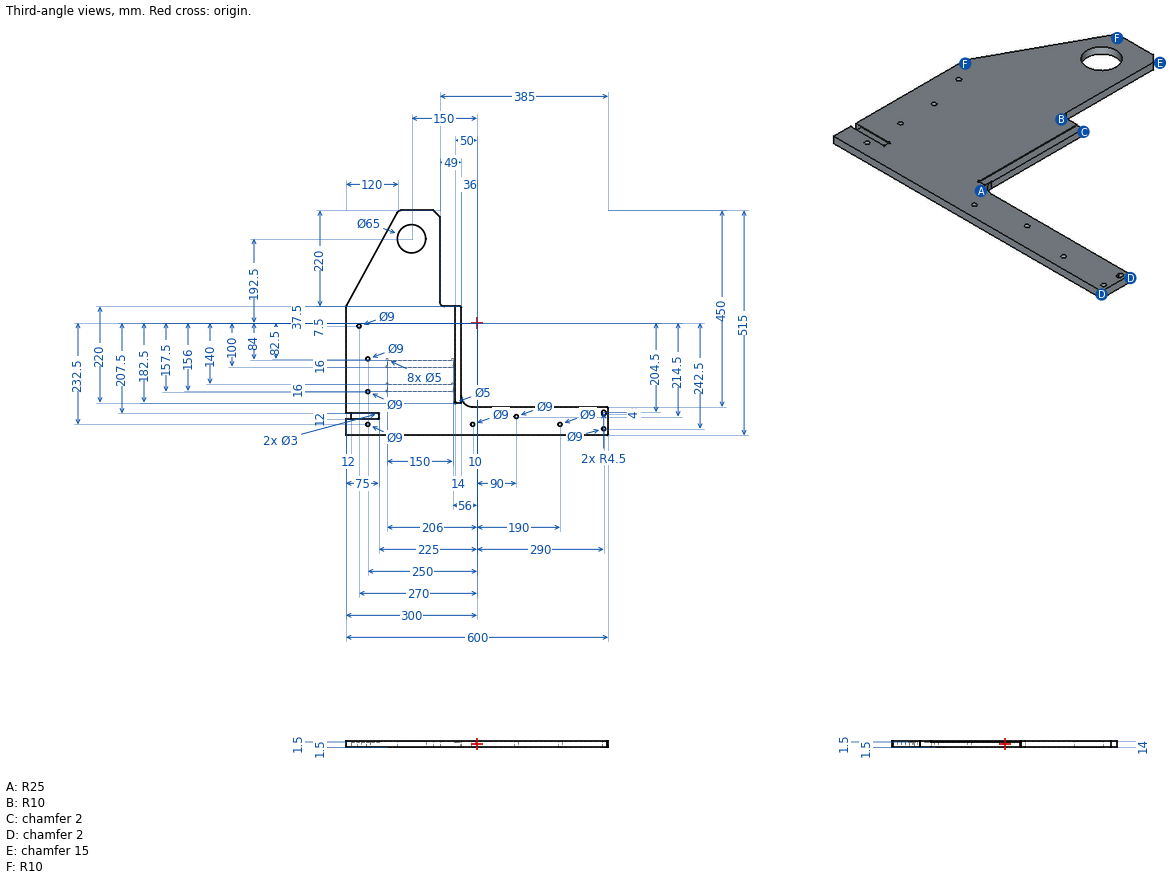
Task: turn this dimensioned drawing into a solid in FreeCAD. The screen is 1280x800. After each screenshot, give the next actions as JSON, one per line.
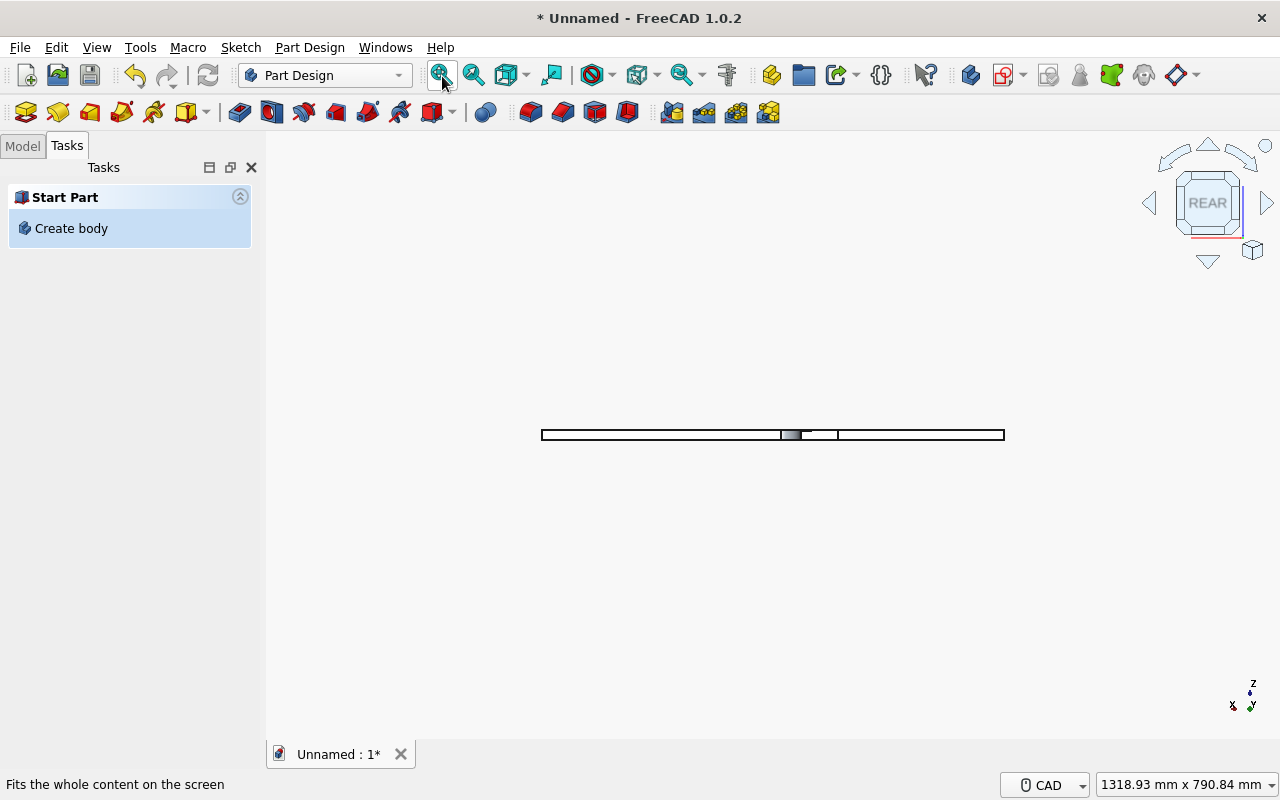
{"action": "scroll", "coordinate": [838, 434], "scroll_direction": "up", "scroll_amount": 7}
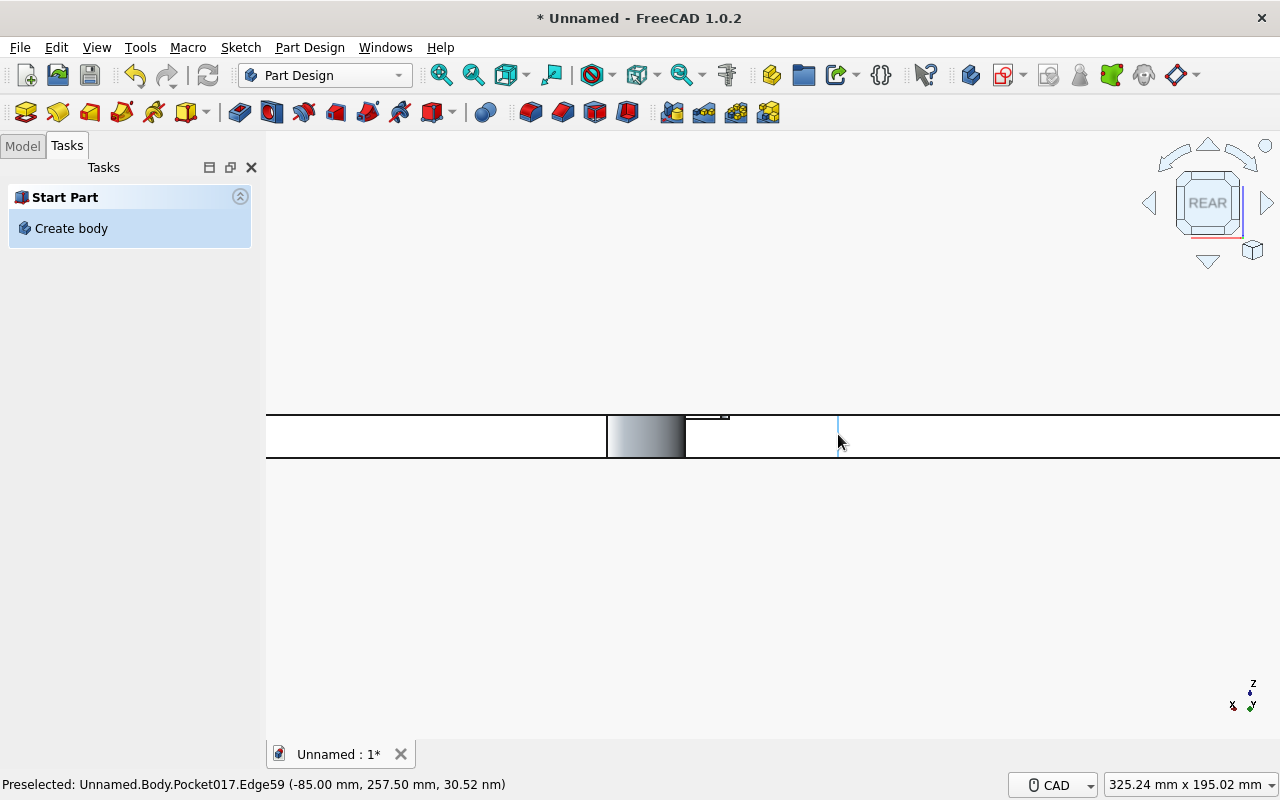
{"action": "left_click", "coordinate": [442, 76]}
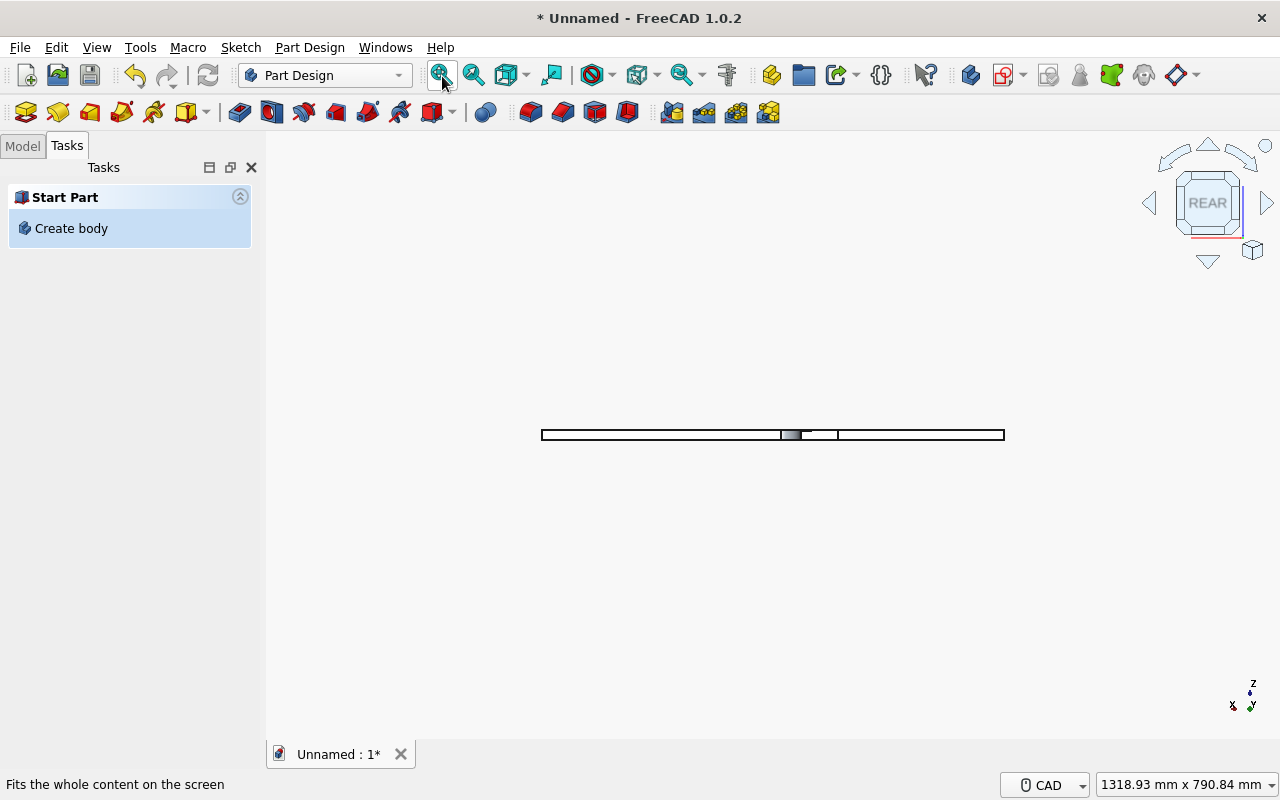
{"action": "key", "text": "6"}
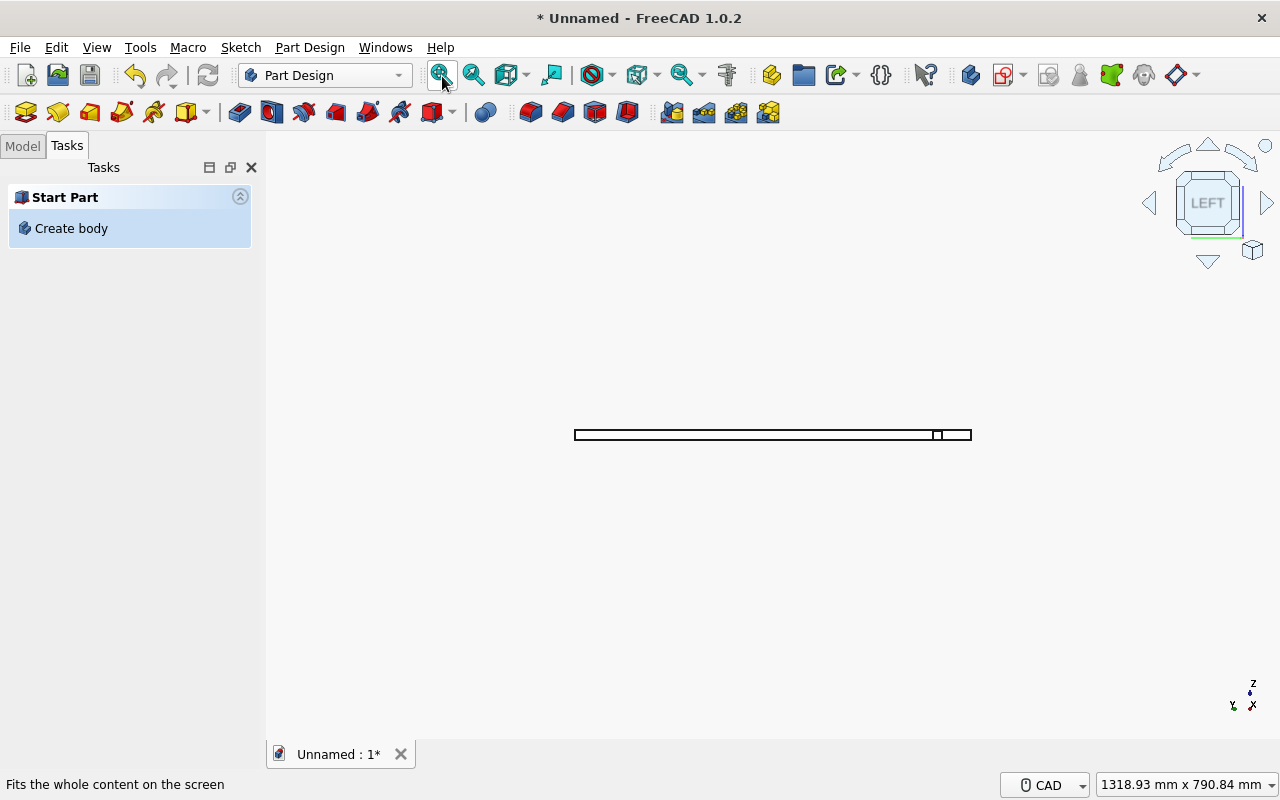
{"action": "left_click", "coordinate": [442, 76]}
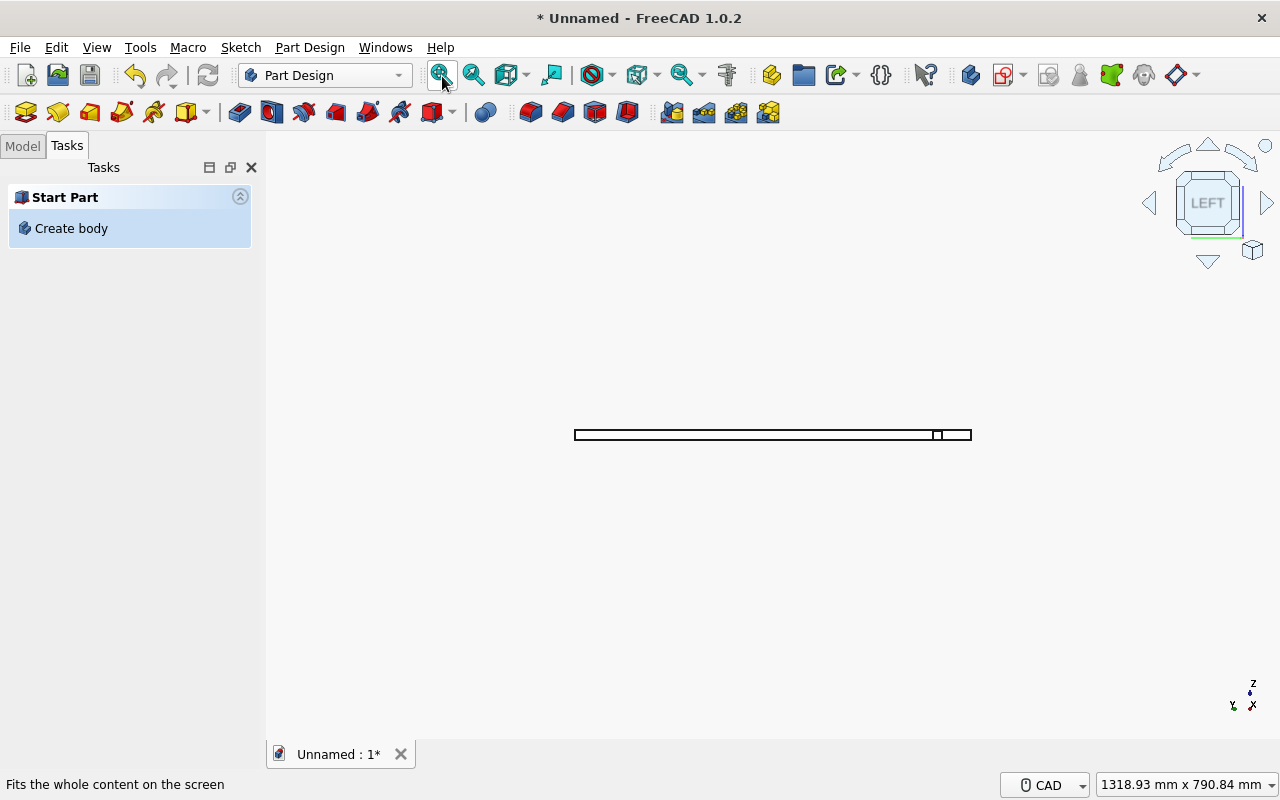
{"action": "scroll", "coordinate": [744, 434], "scroll_direction": "up", "scroll_amount": 7}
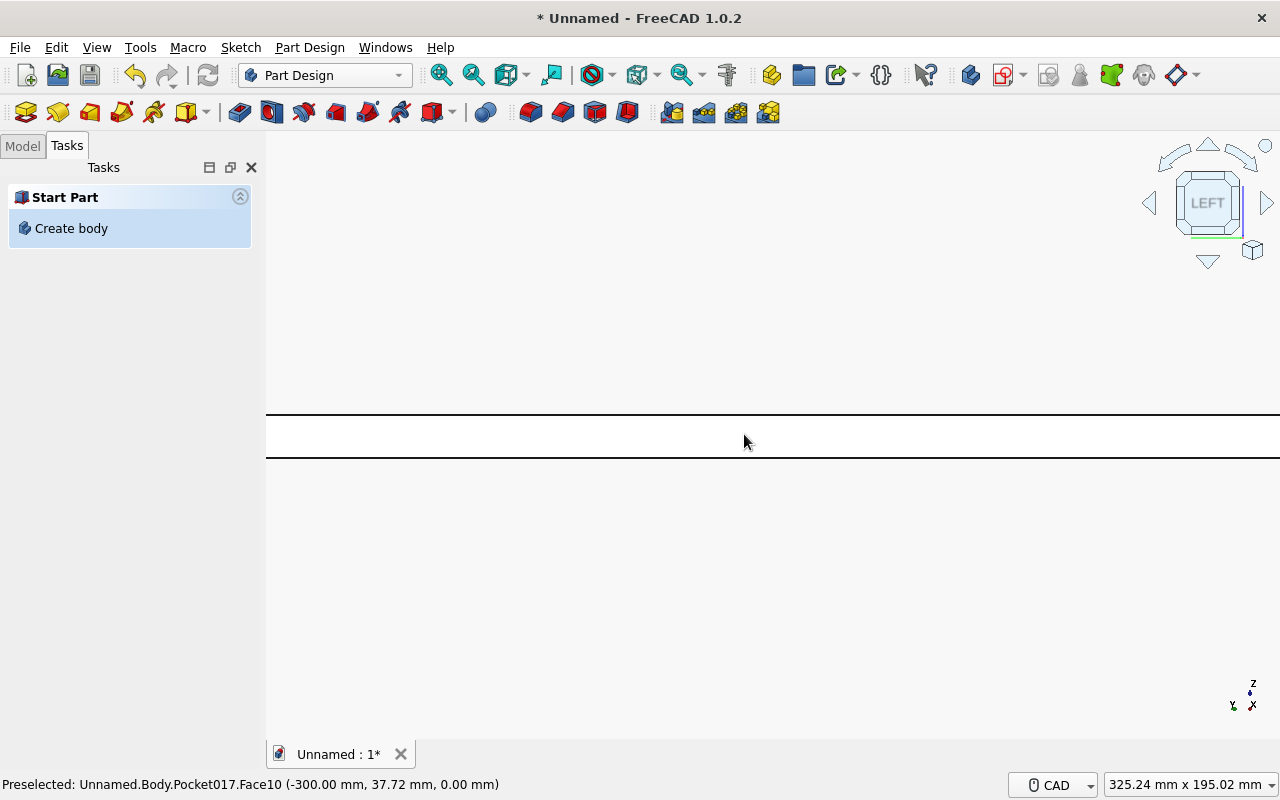
{"action": "left_click", "coordinate": [442, 76]}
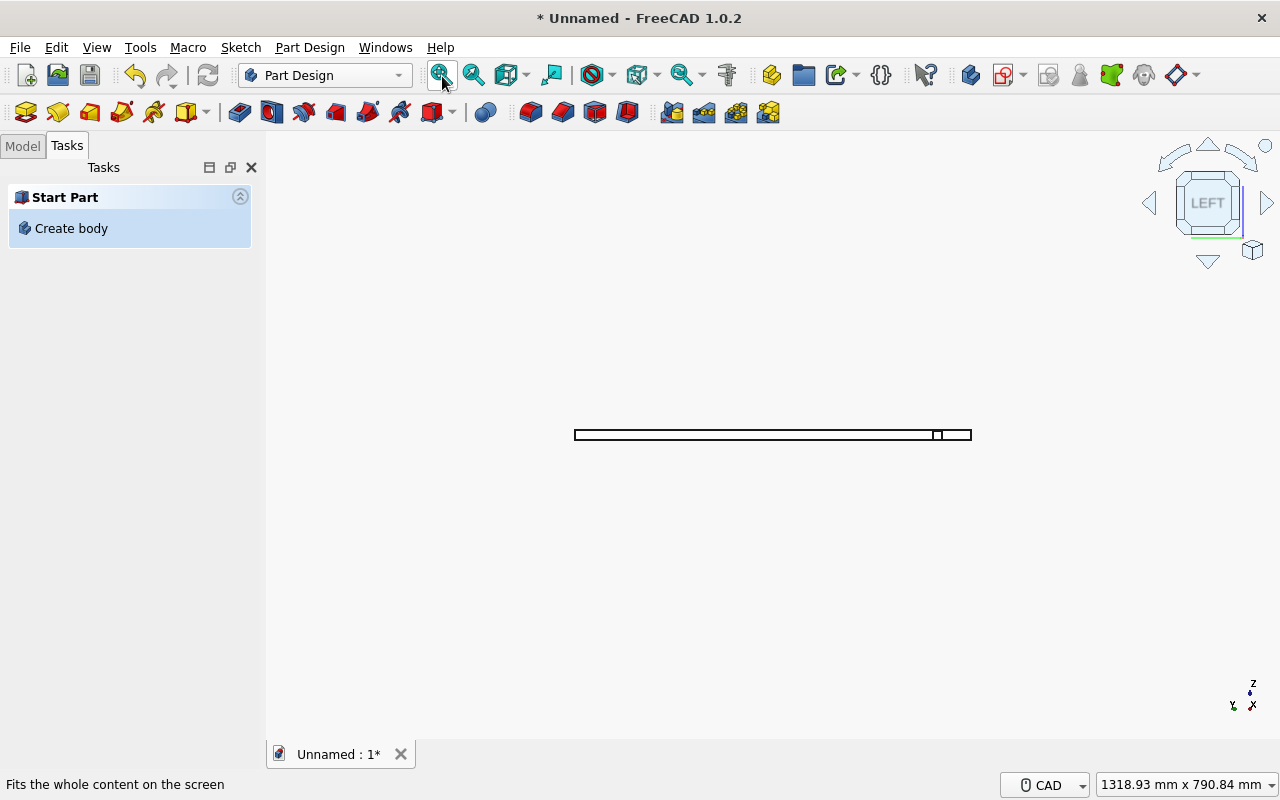
{"action": "key", "text": "v 3"}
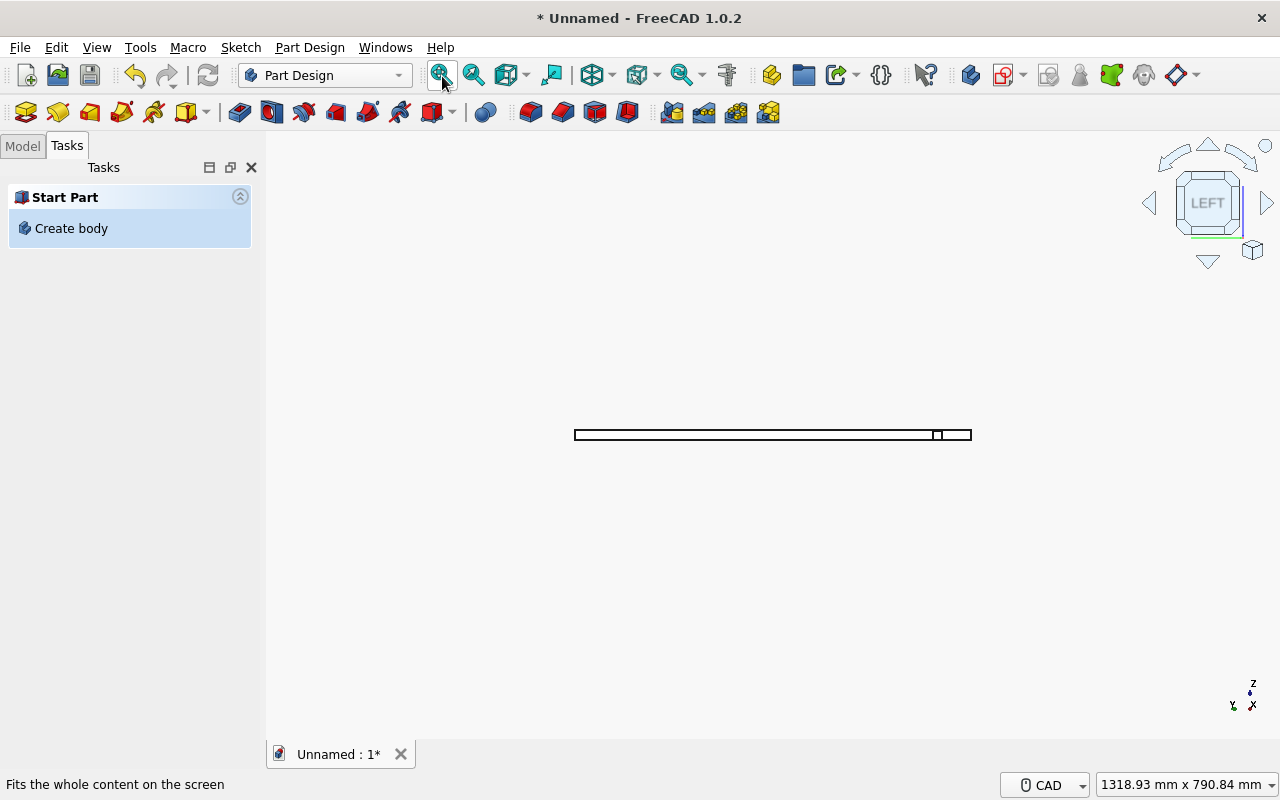
{"action": "key", "text": "0"}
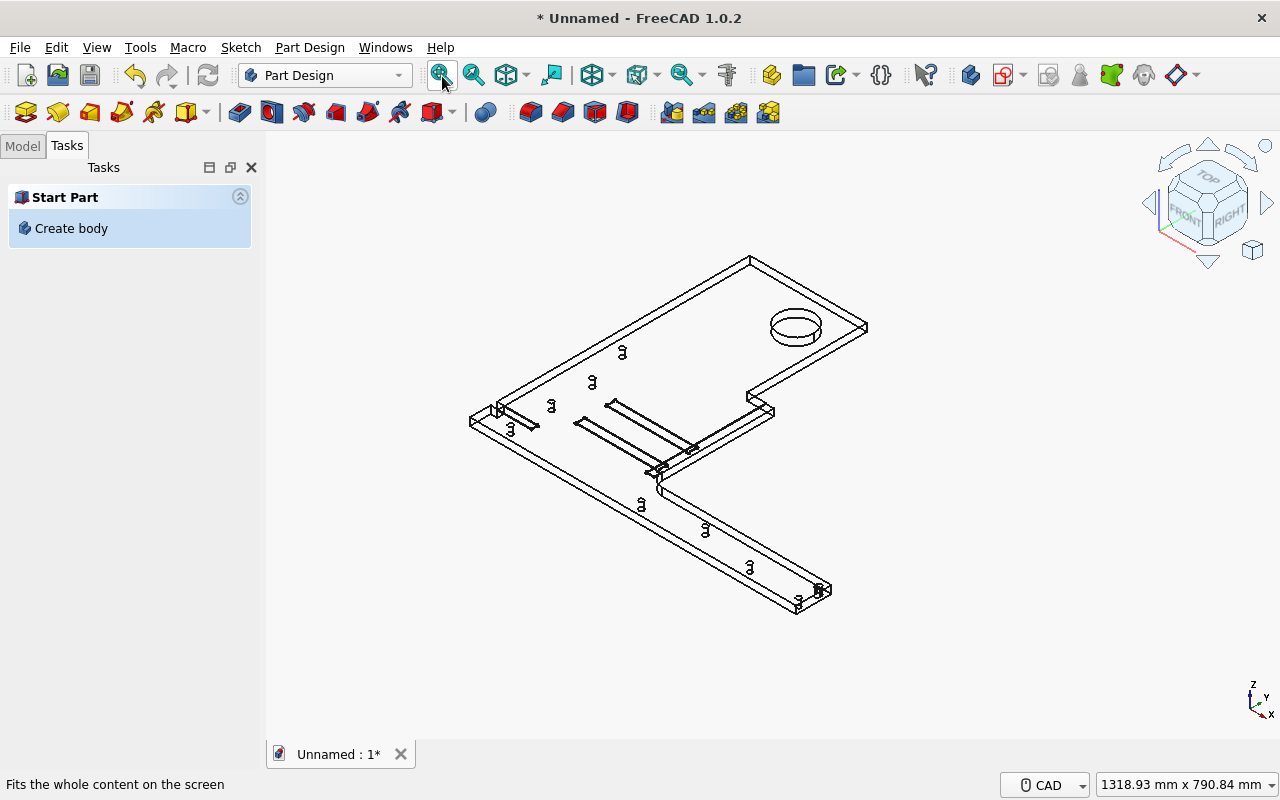
{"action": "scroll", "coordinate": [747, 396], "scroll_direction": "up", "scroll_amount": 7}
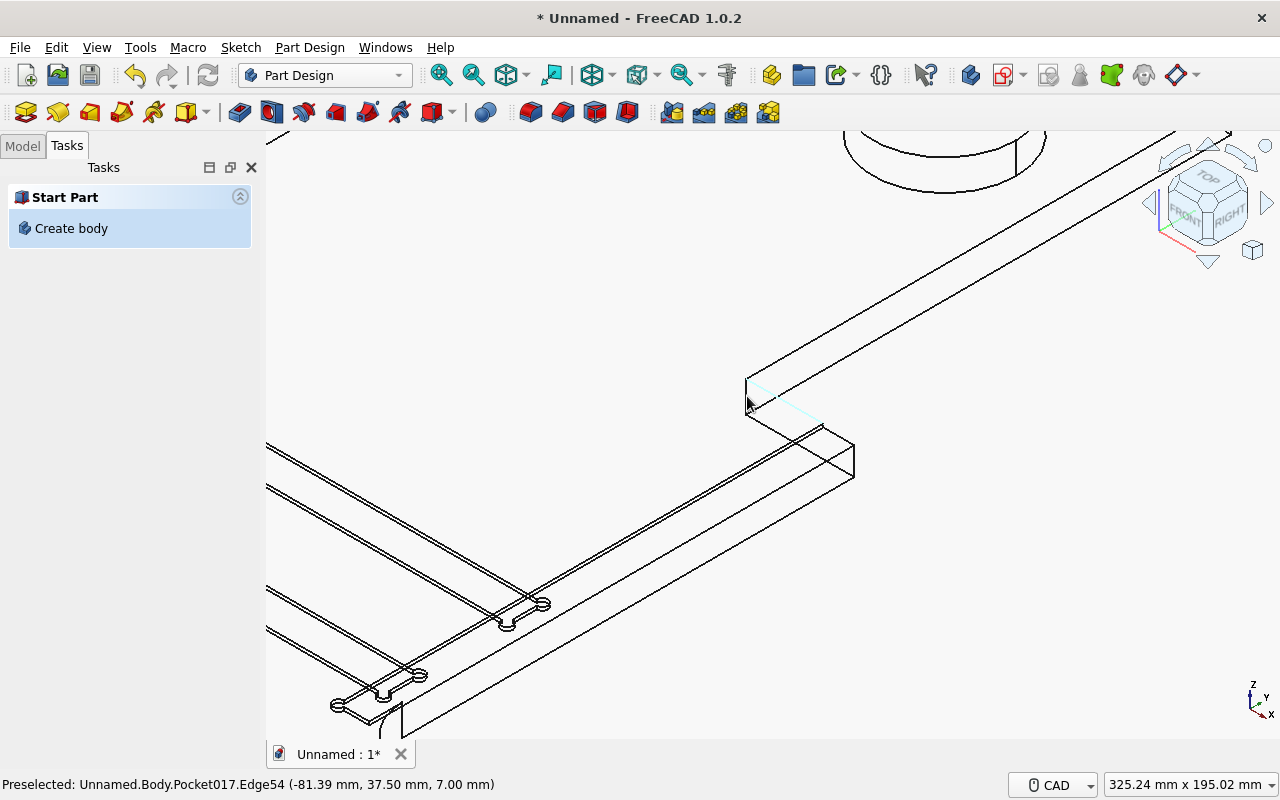
{"action": "left_click", "coordinate": [746, 396]}